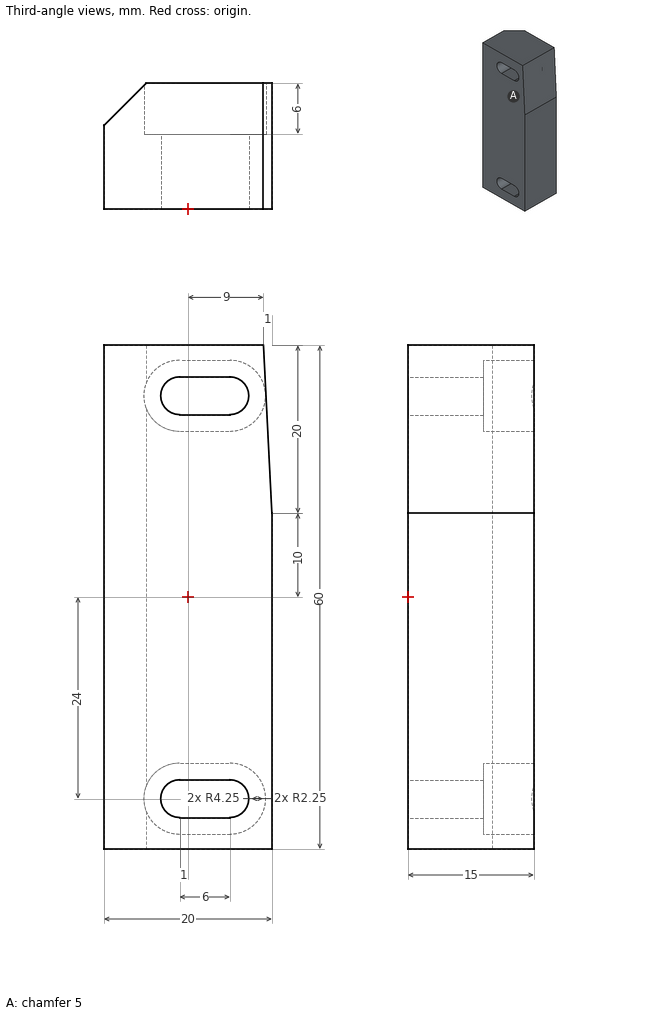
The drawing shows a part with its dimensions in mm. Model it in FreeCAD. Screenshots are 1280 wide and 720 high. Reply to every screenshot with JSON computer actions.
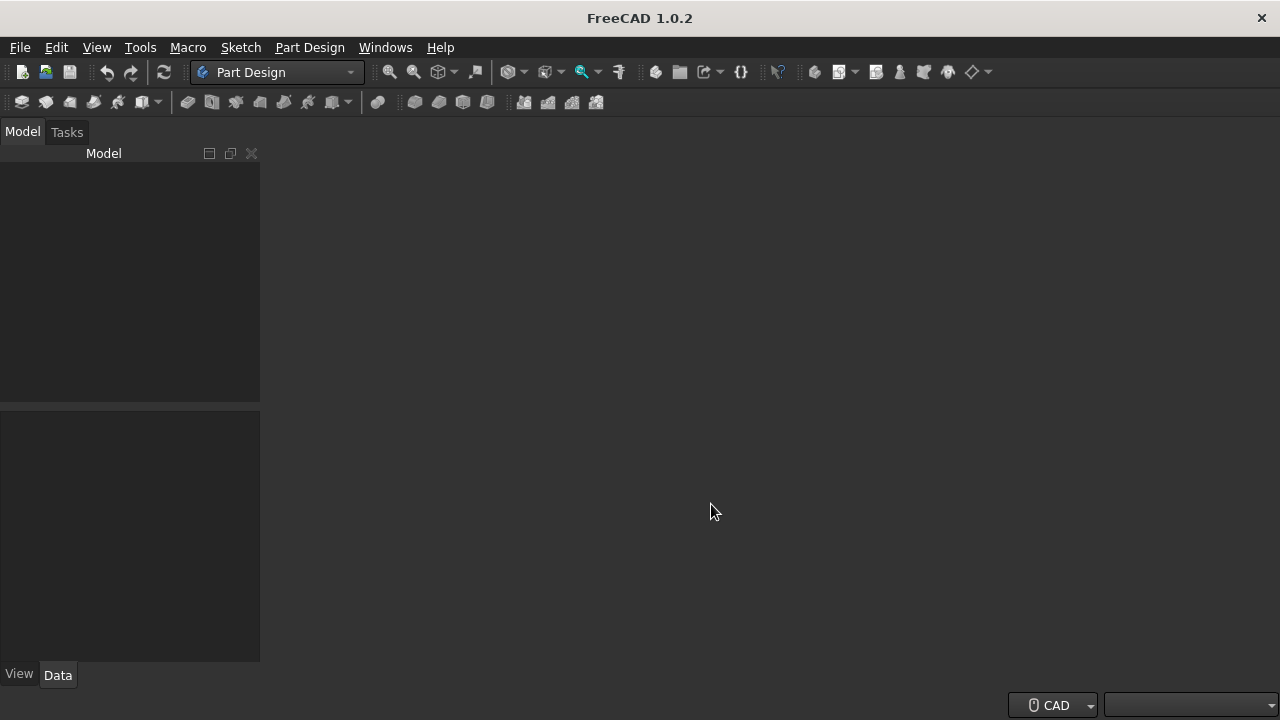
{"action": "left_click", "coordinate": [22, 72]}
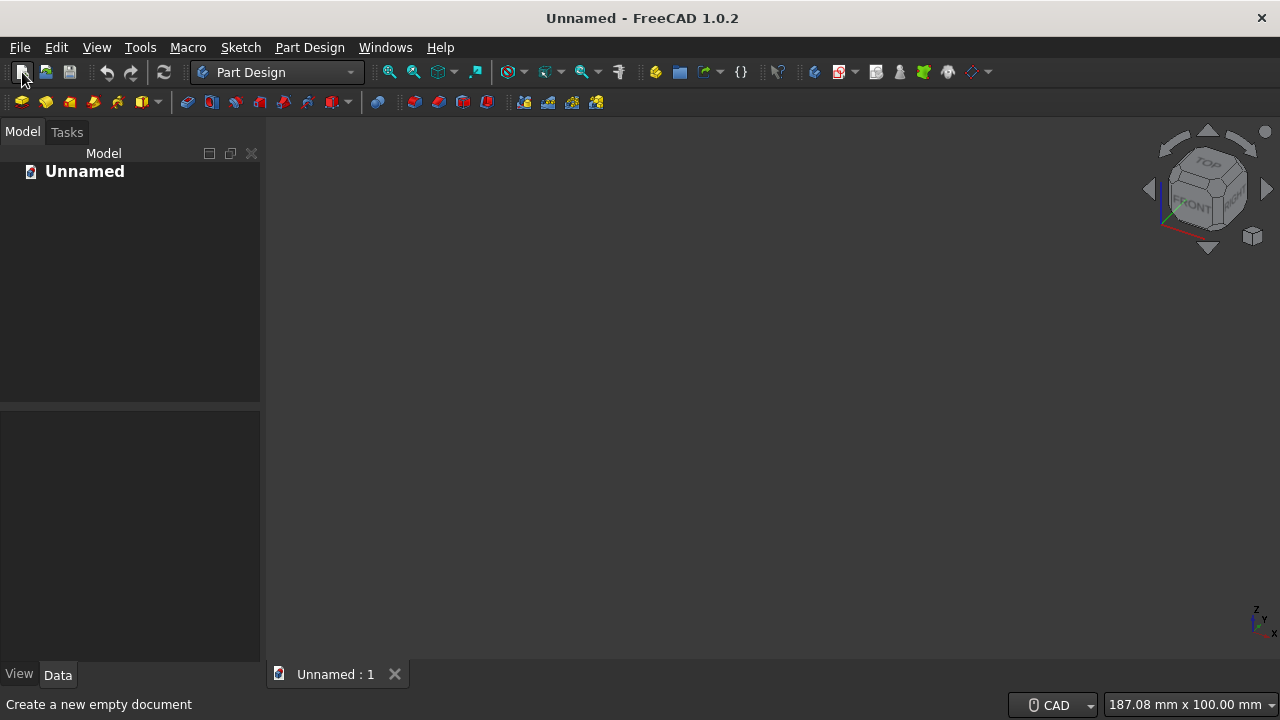
{"action": "left_click", "coordinate": [840, 72]}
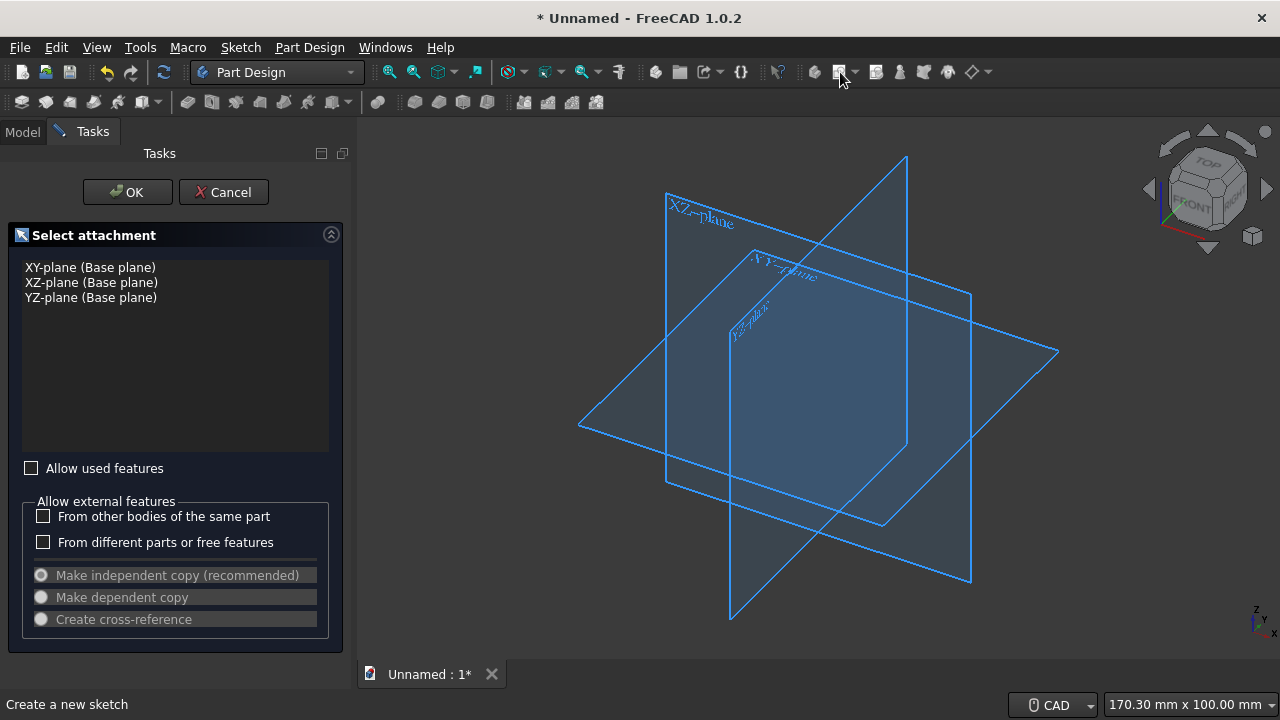
{"action": "left_click", "coordinate": [82, 282]}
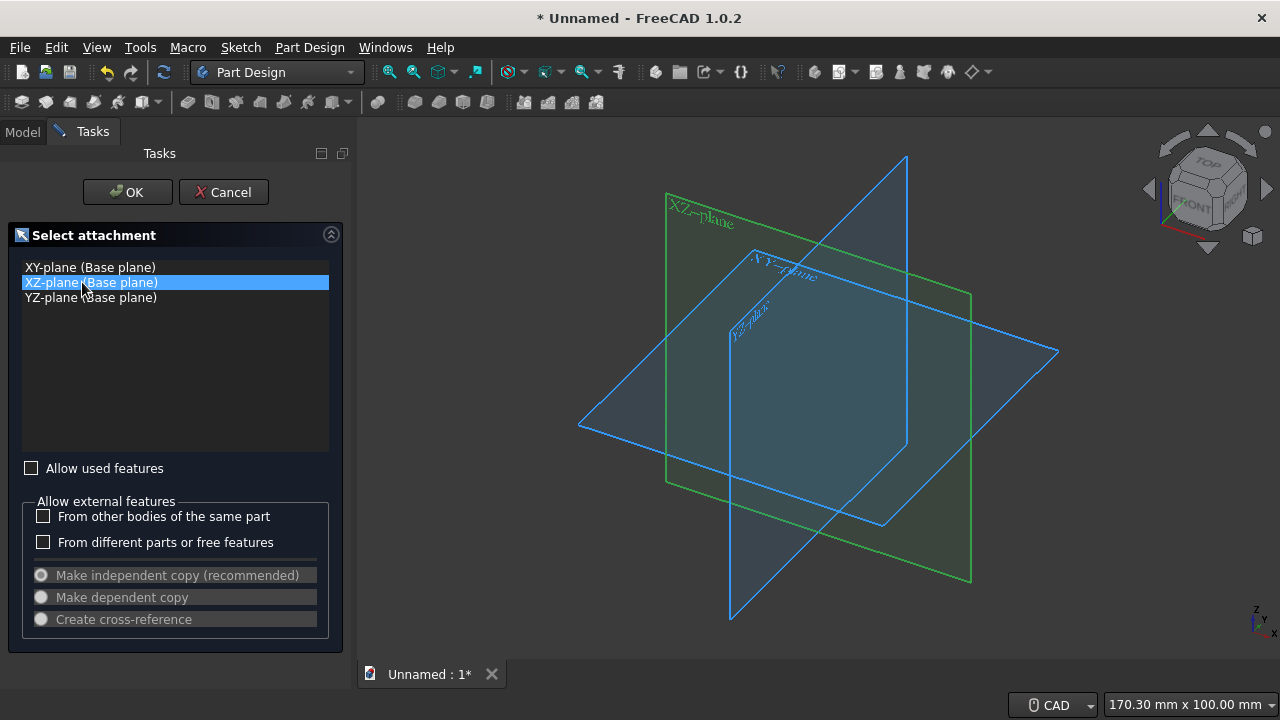
{"action": "left_click", "coordinate": [128, 192]}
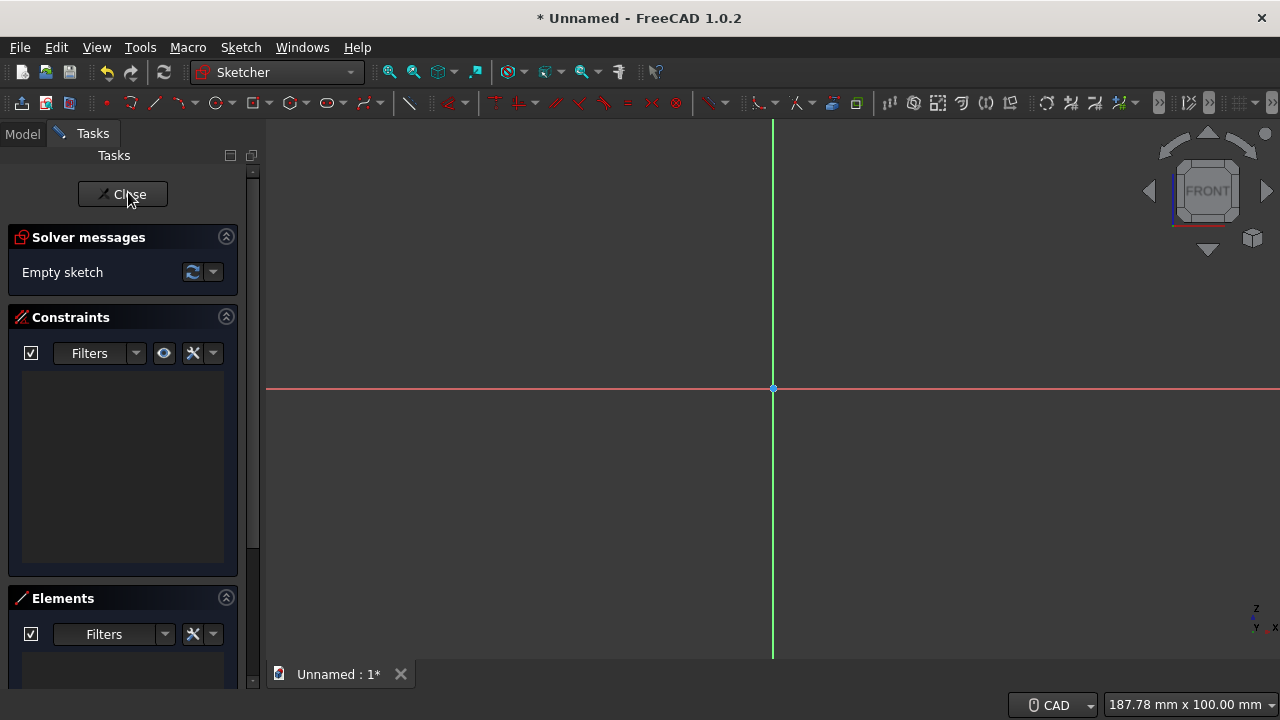
{"action": "left_click", "coordinate": [254, 104]}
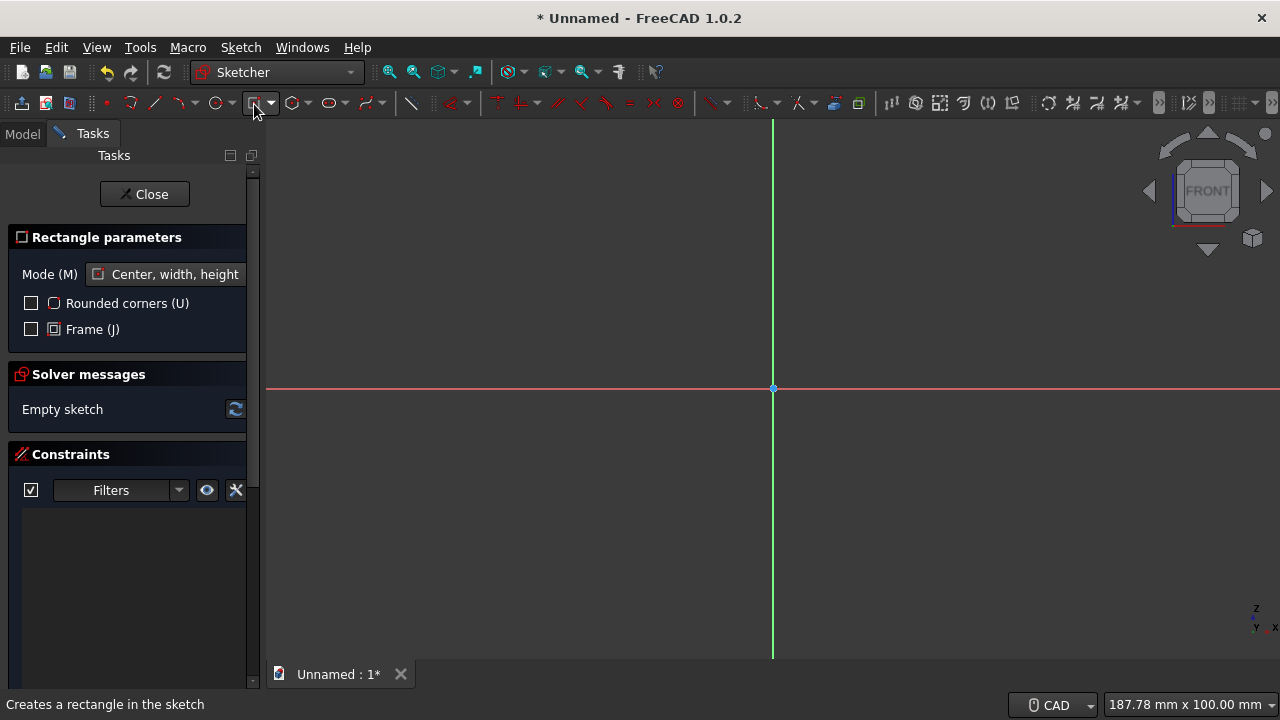
{"action": "left_click", "coordinate": [773, 389]}
{"action": "left_click", "coordinate": [827, 227]}
{"action": "key", "text": "Escape"}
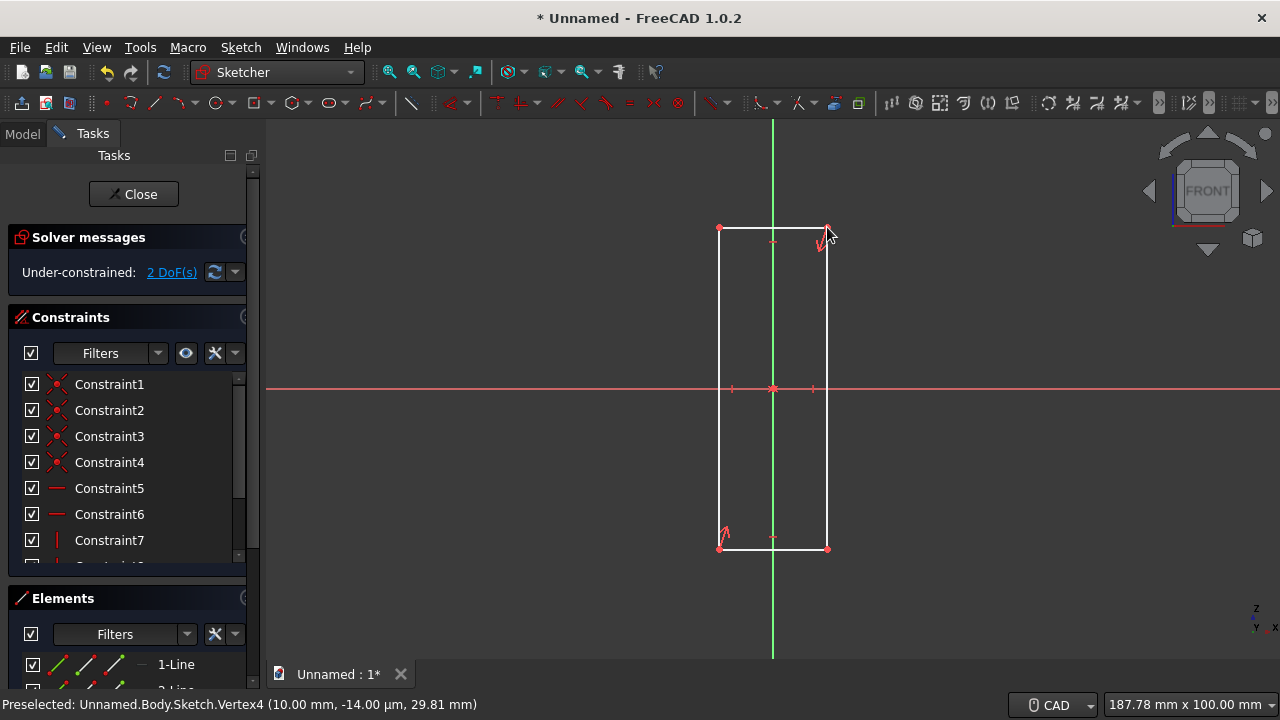
{"action": "left_click", "coordinate": [450, 104]}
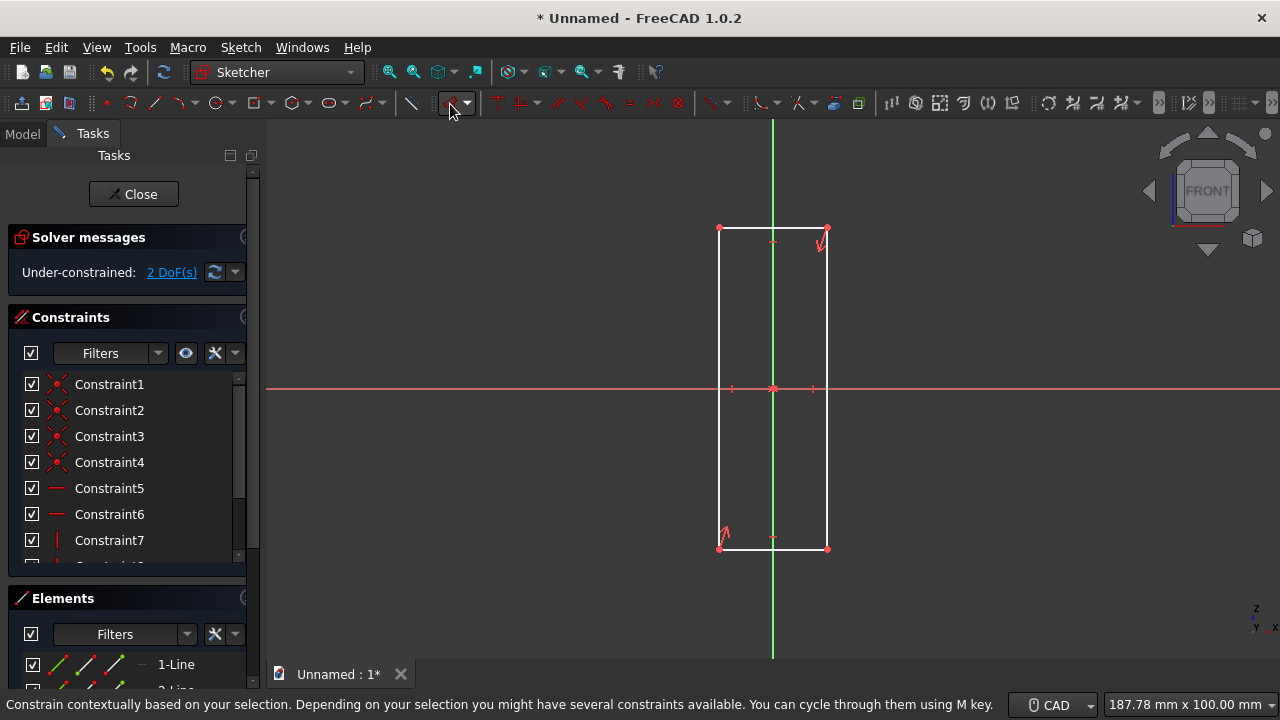
{"action": "left_click", "coordinate": [751, 550]}
{"action": "left_click", "coordinate": [748, 584]}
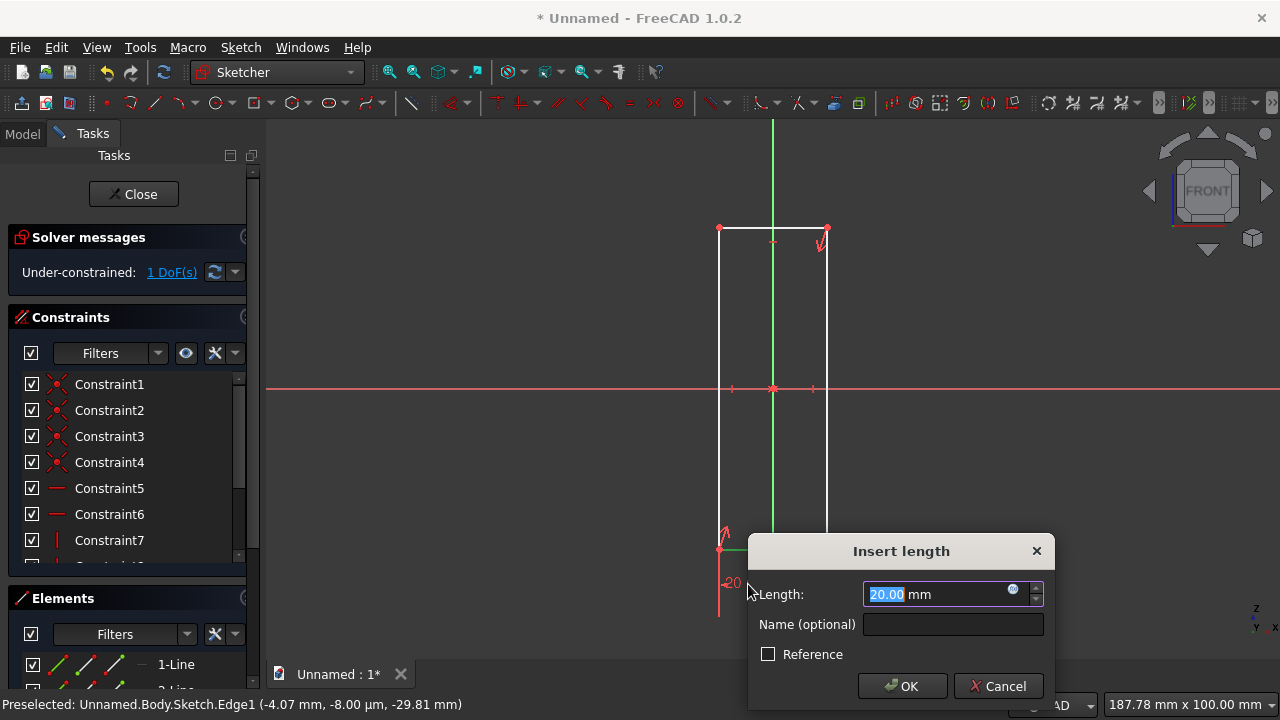
{"action": "type", "text": "20"}
{"action": "key", "text": "Return"}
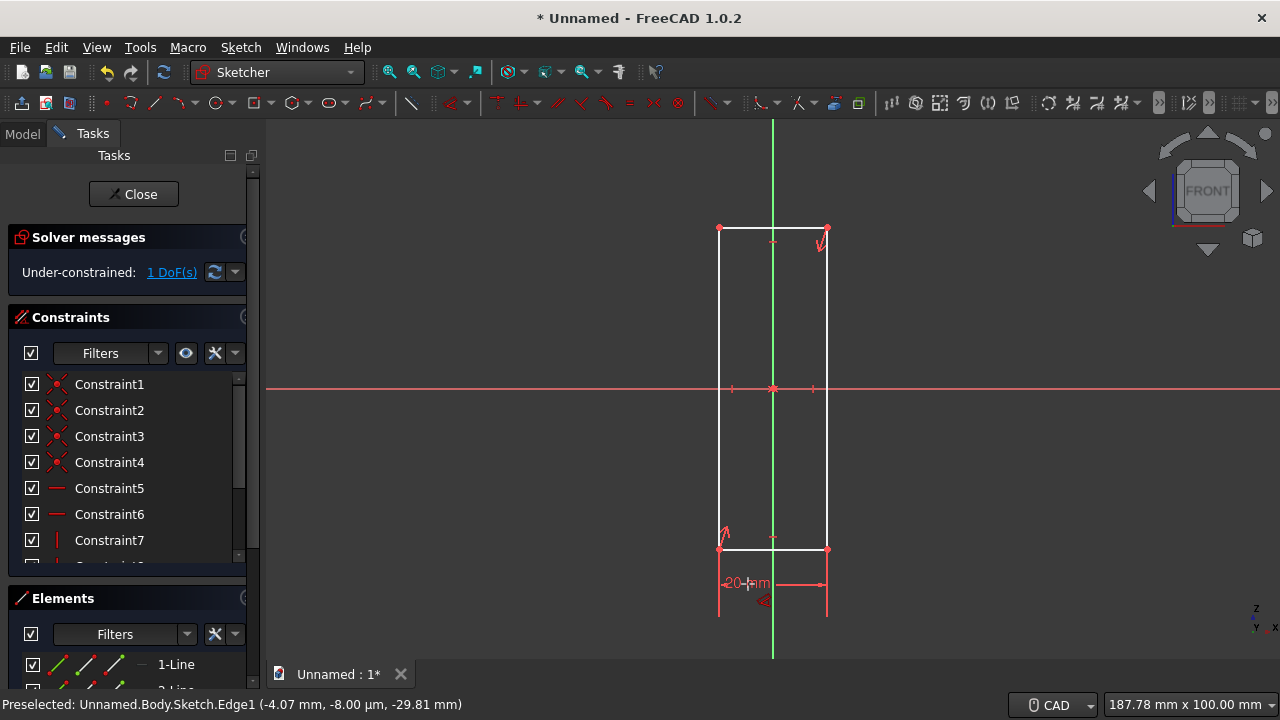
{"action": "left_click", "coordinate": [827, 453]}
{"action": "left_click", "coordinate": [861, 315]}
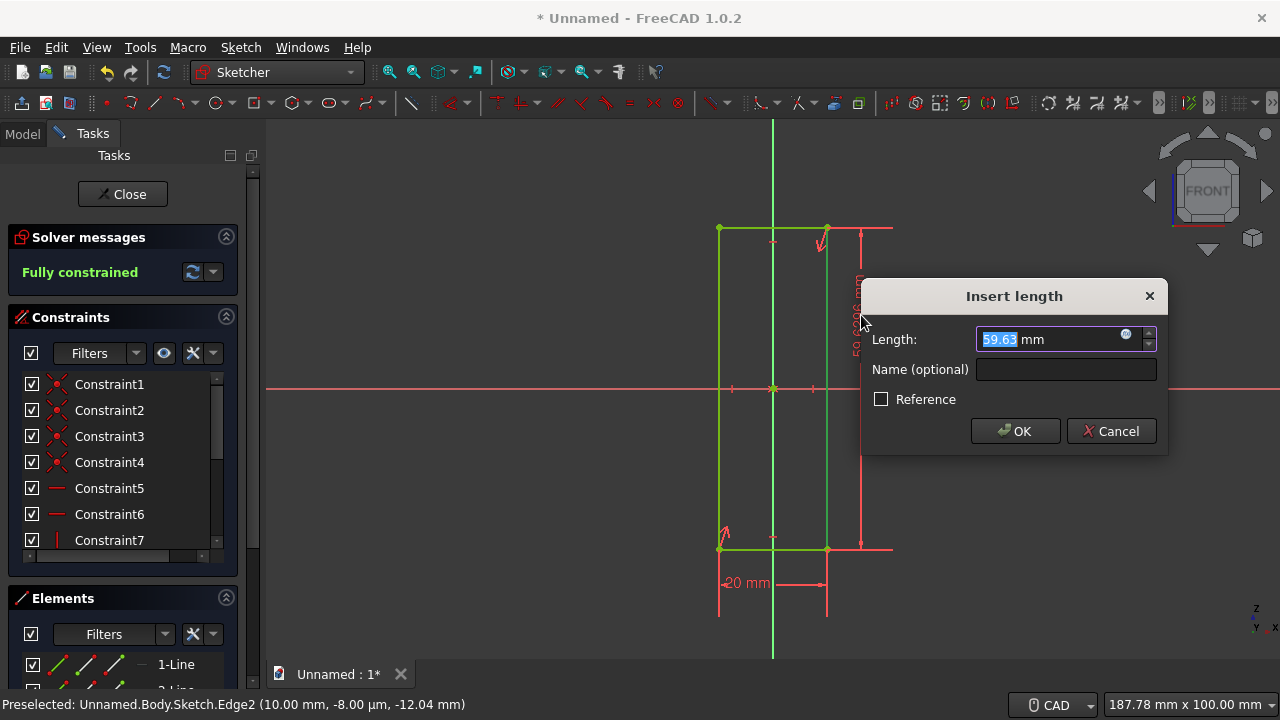
{"action": "type", "text": "60"}
{"action": "key", "text": "Return"}
{"action": "key", "text": "Escape"}